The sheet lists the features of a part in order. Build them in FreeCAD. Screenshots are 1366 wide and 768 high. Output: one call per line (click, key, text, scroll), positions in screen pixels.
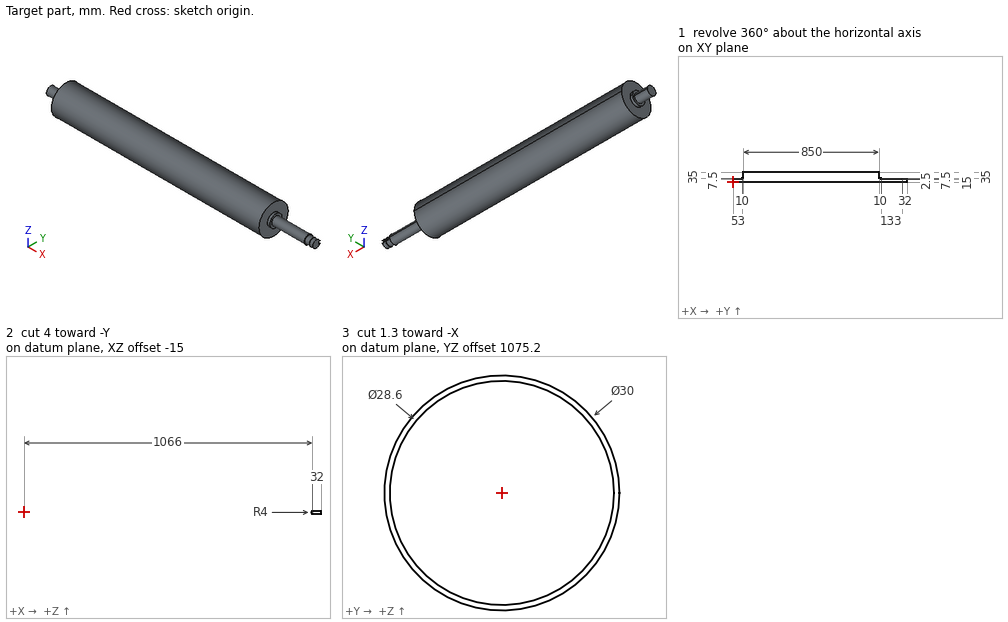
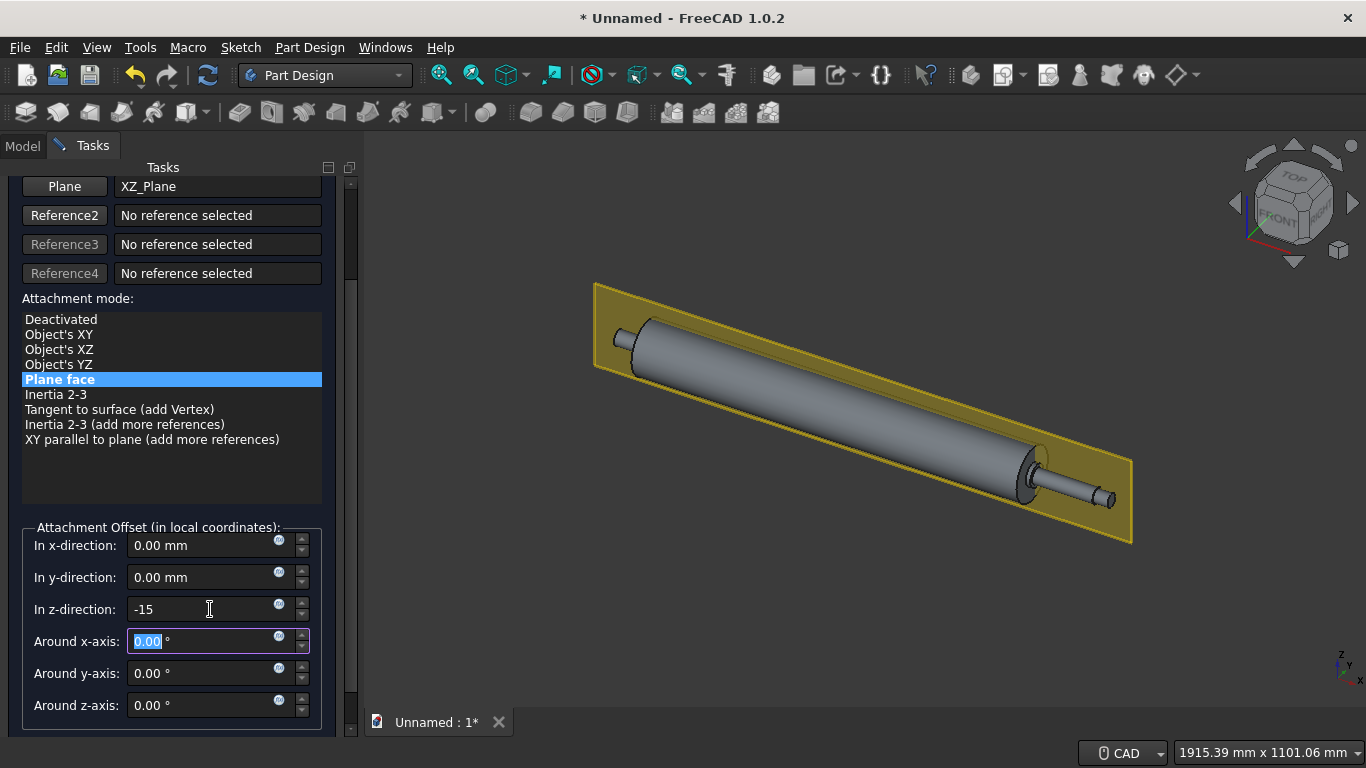
scroll(351, 456, up, 3)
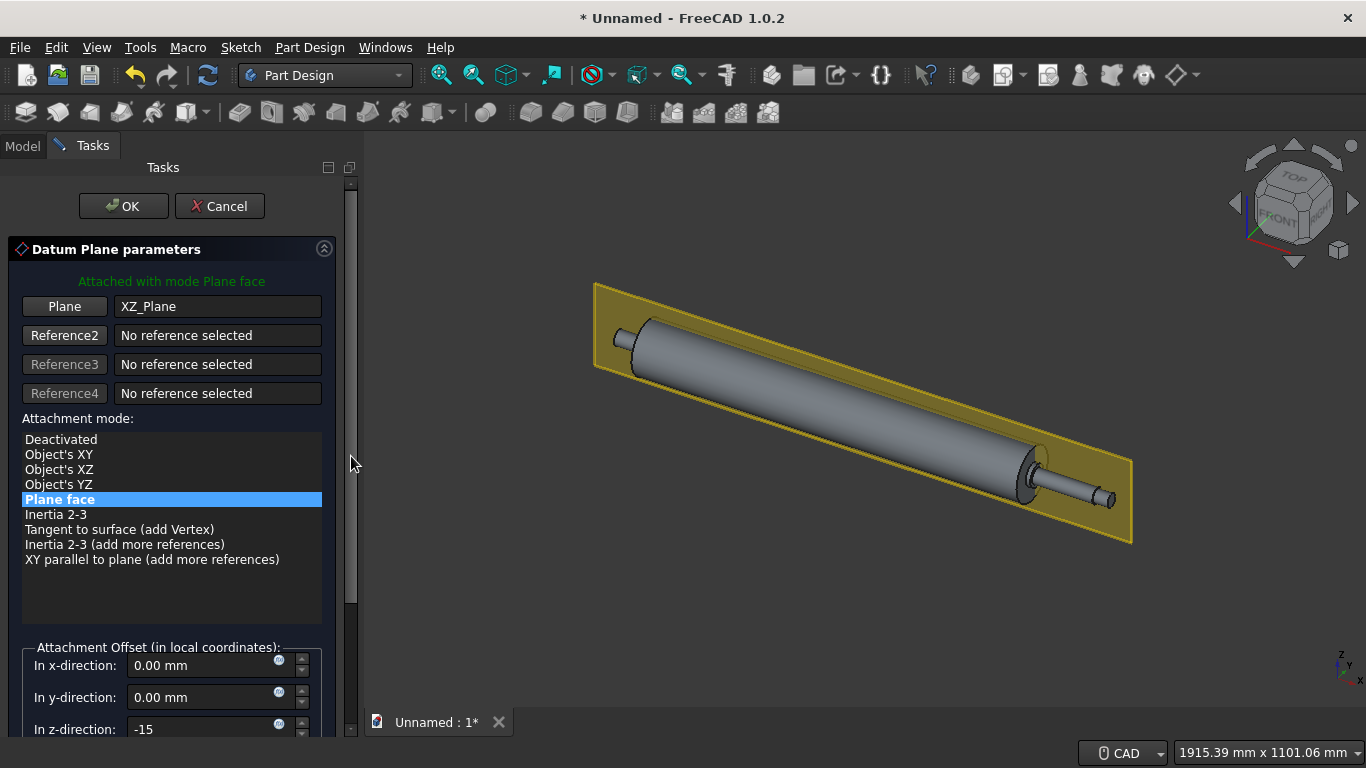
click(124, 206)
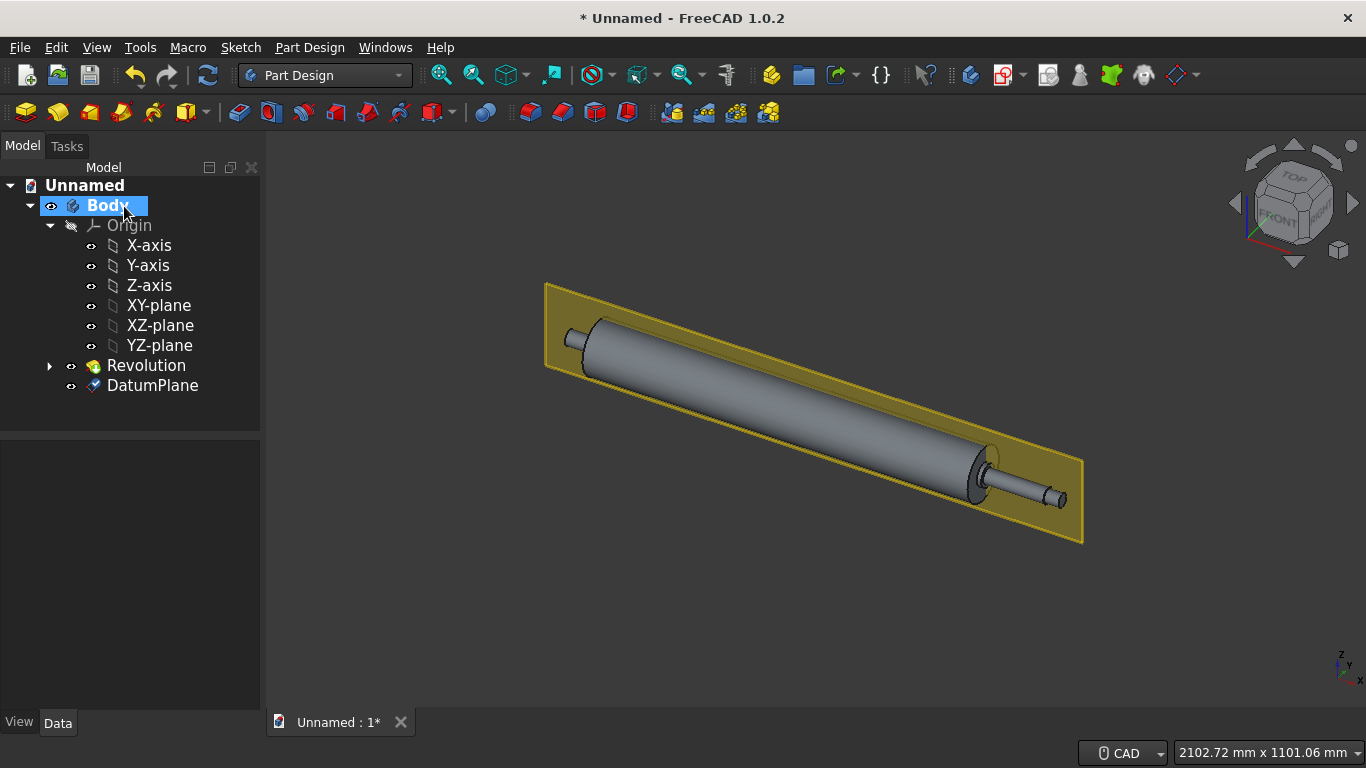
click(116, 386)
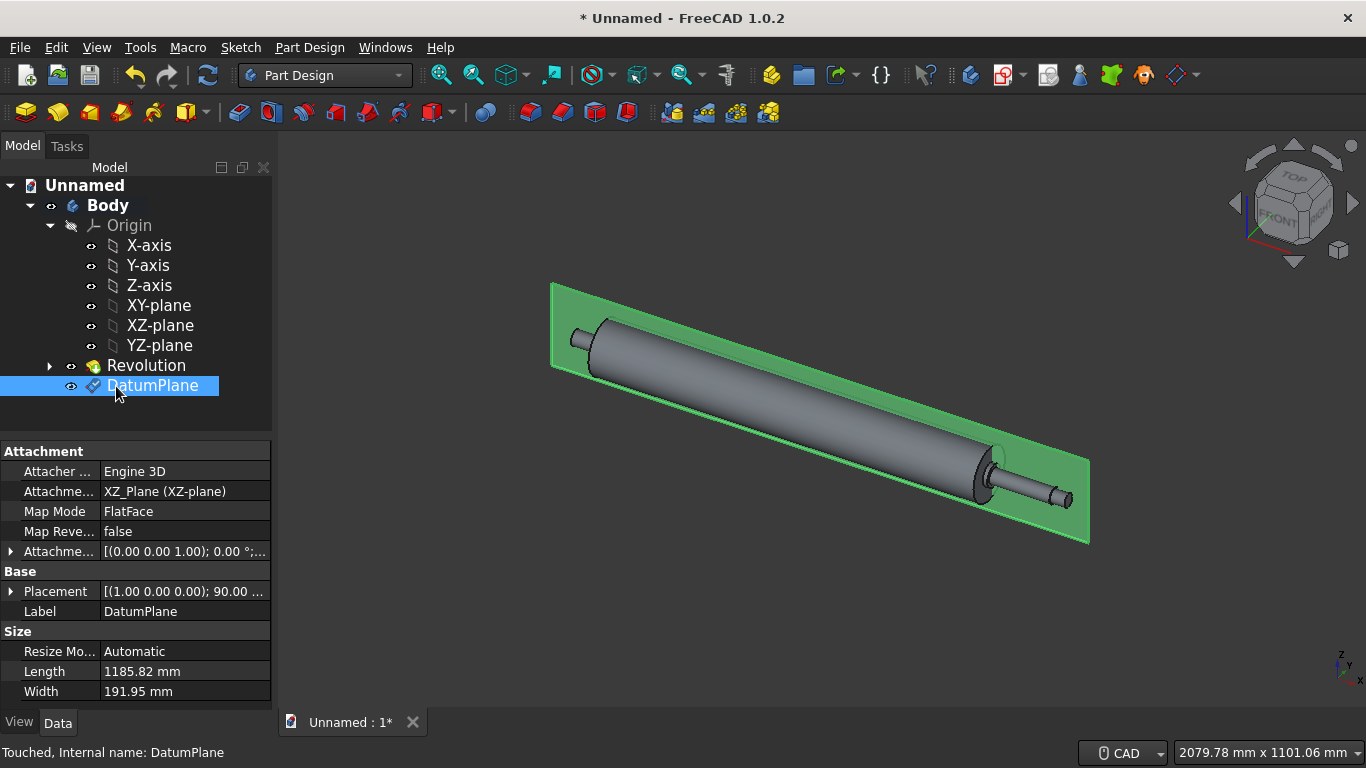
click(1004, 76)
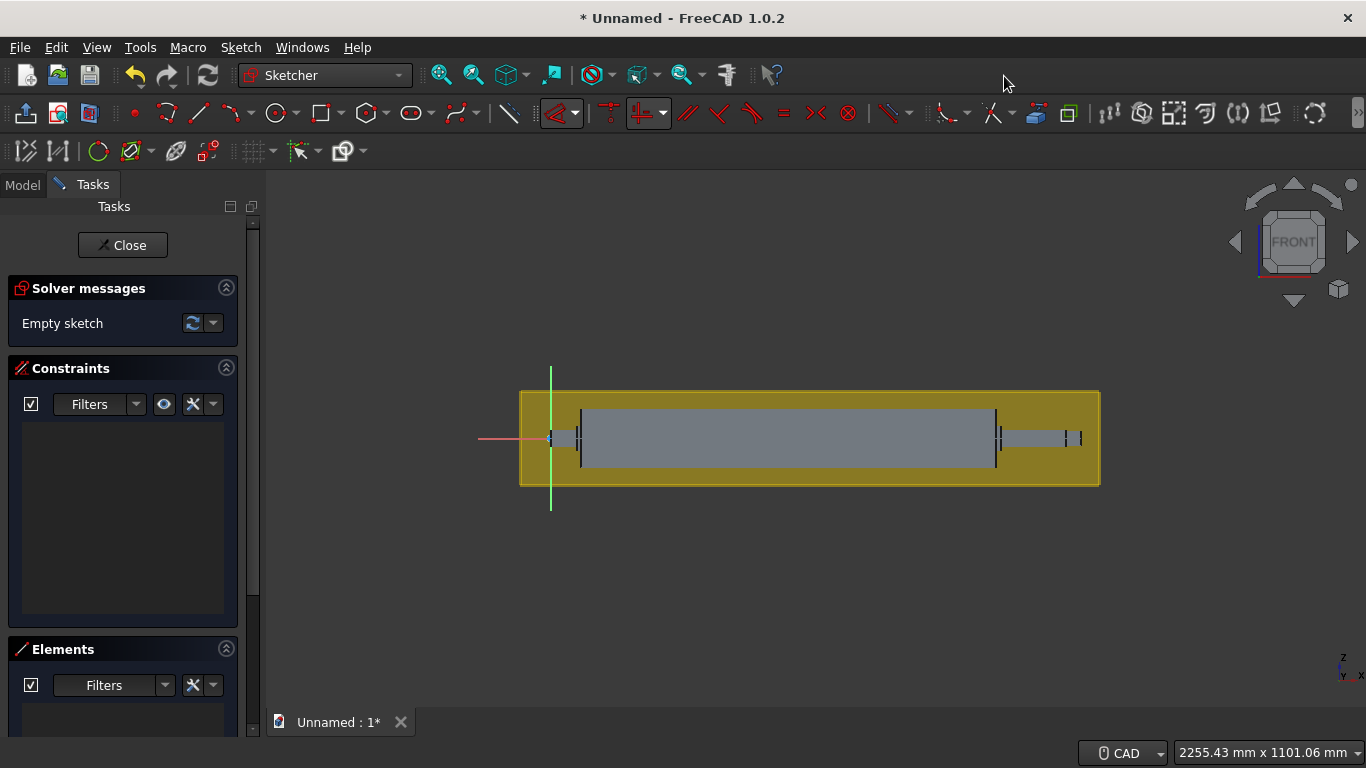
click(90, 114)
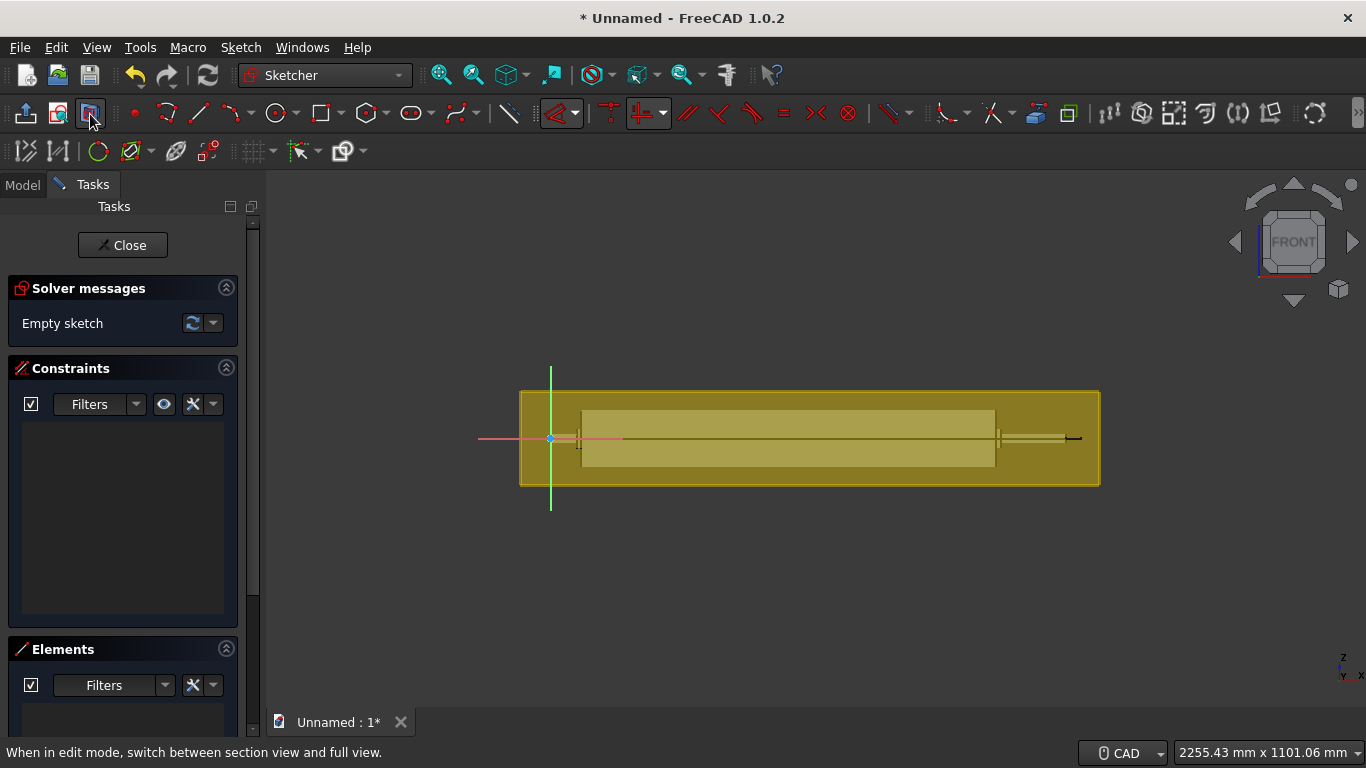
scroll(1095, 438, up, 15)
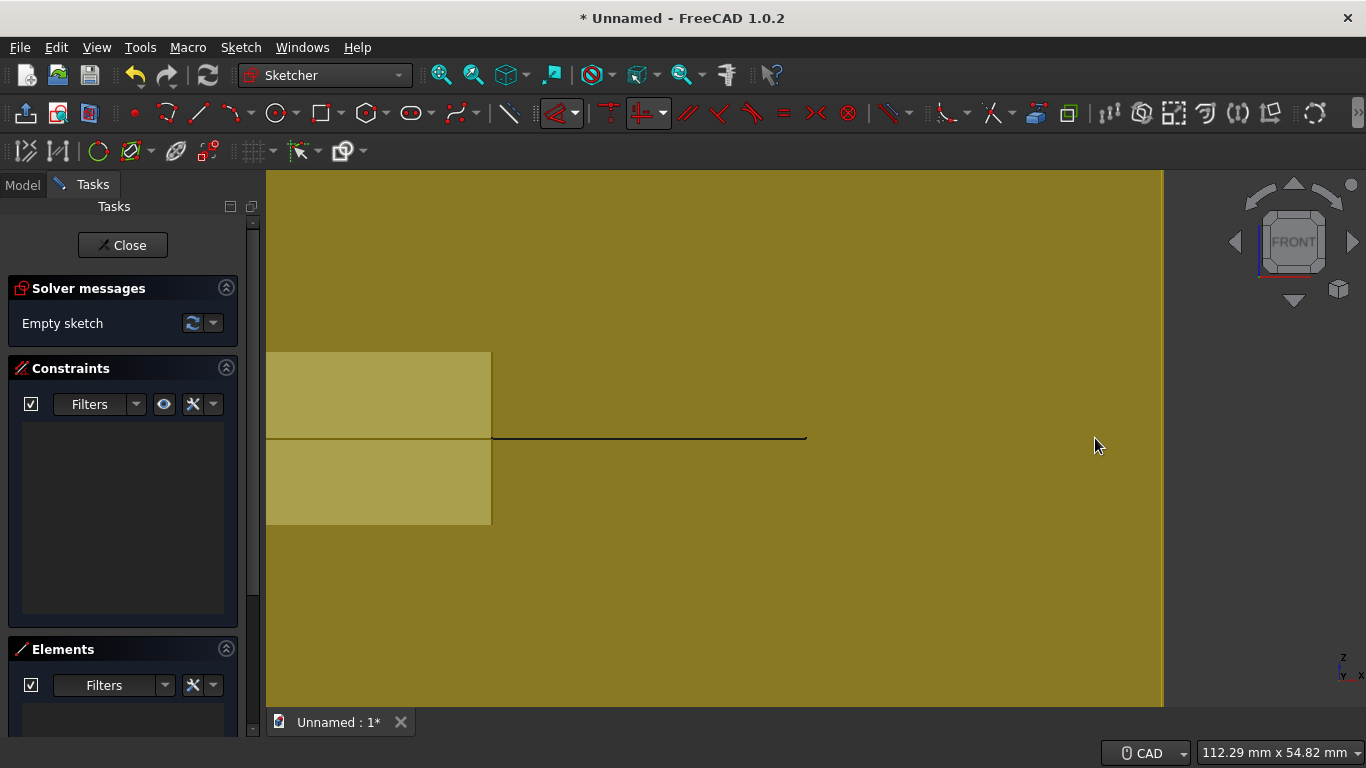
scroll(703, 439, up, 3)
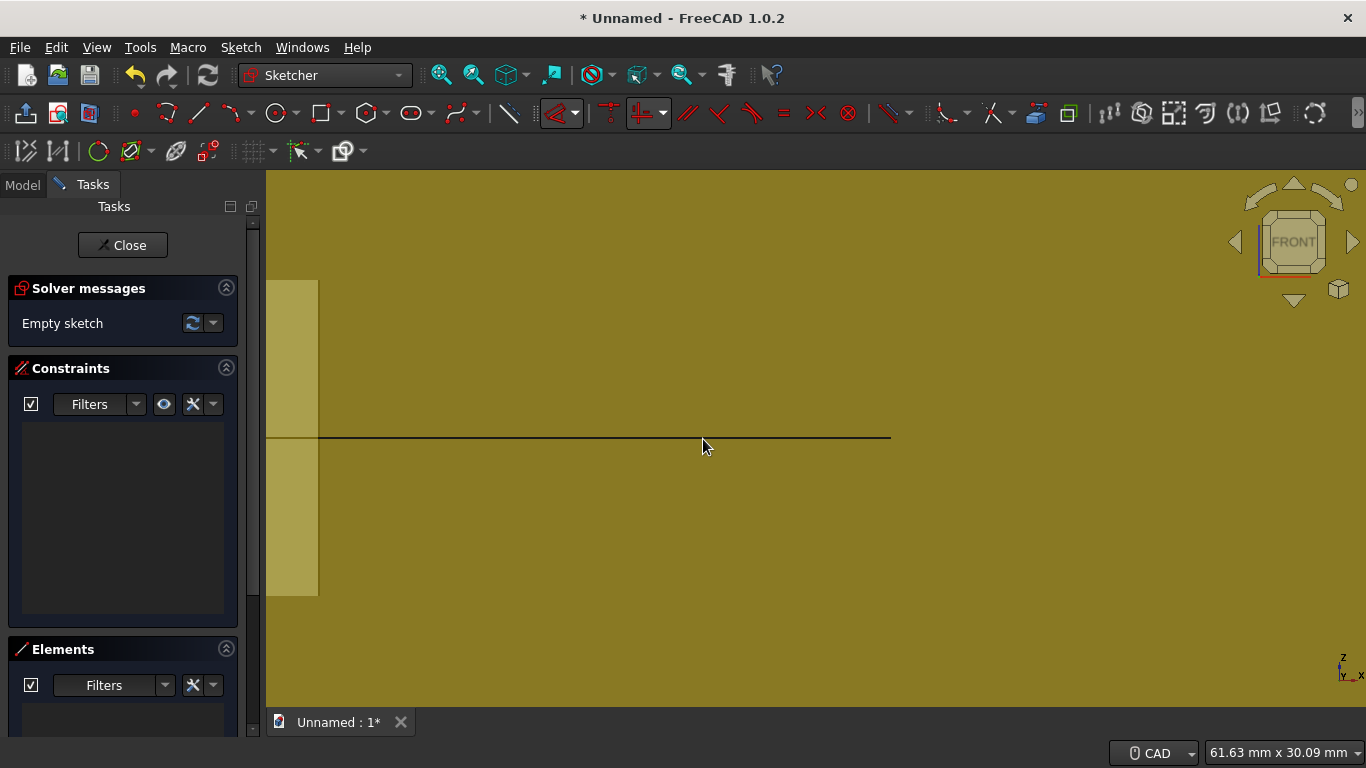
click(168, 114)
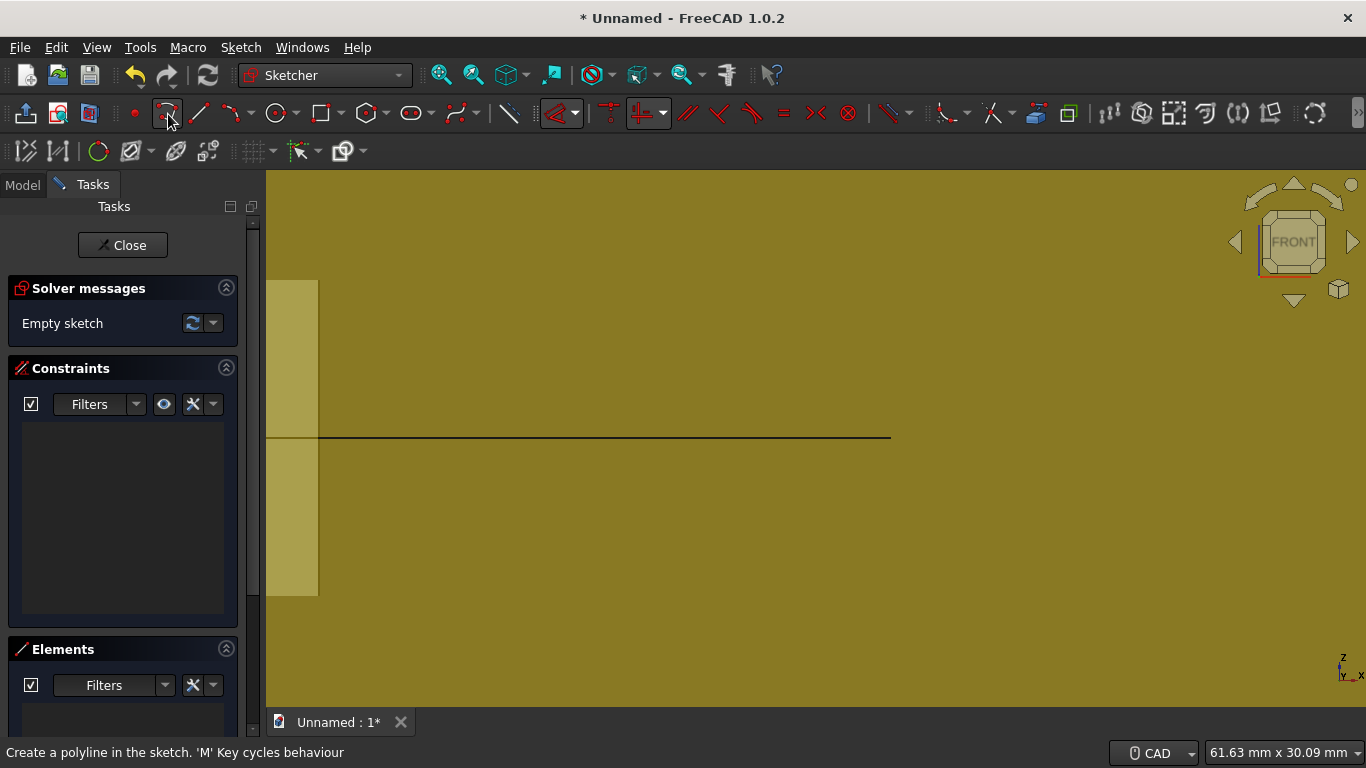
click(497, 366)
click(1068, 366)
click(1068, 509)
click(497, 509)
right_click(497, 509)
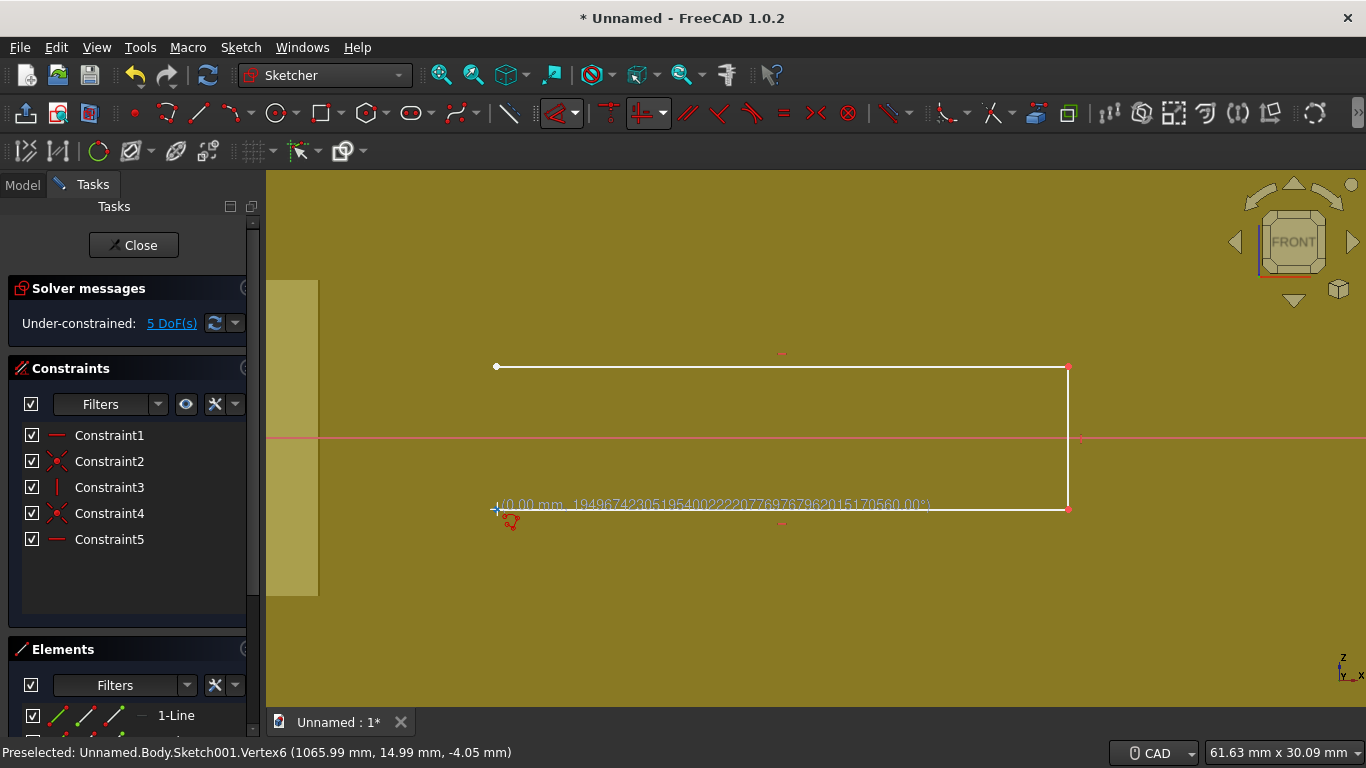
click(232, 114)